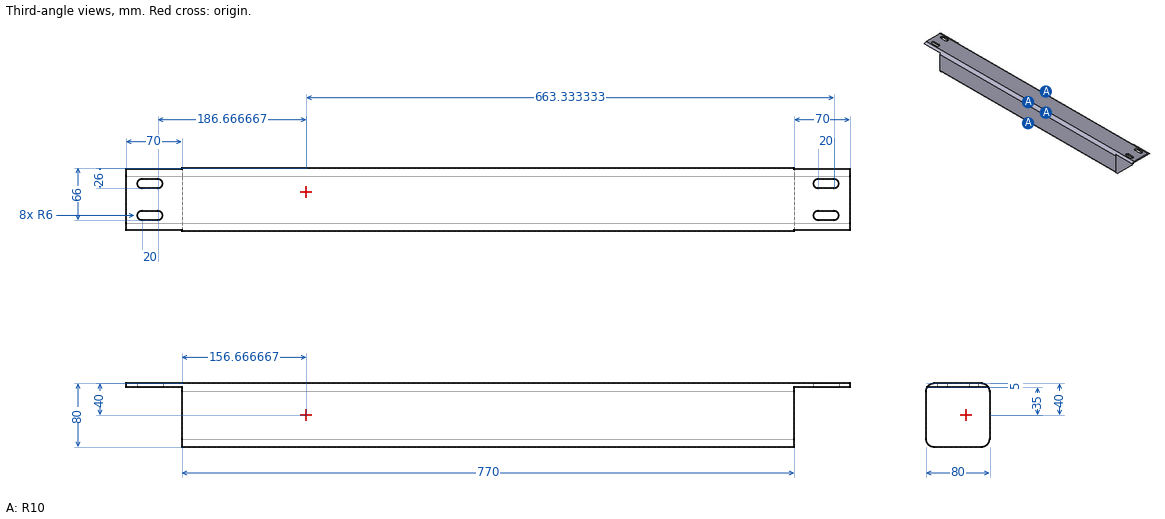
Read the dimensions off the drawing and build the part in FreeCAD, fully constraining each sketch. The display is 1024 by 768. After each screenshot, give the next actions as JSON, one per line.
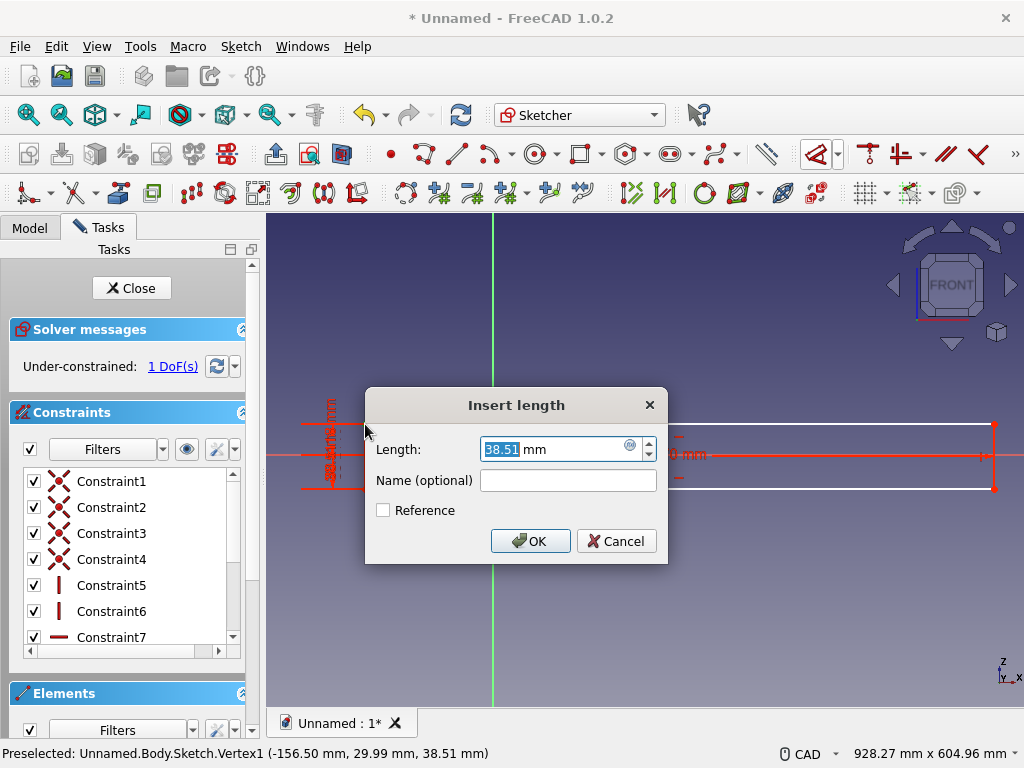
{"action": "type", "text": "40"}
{"action": "key", "text": "Return"}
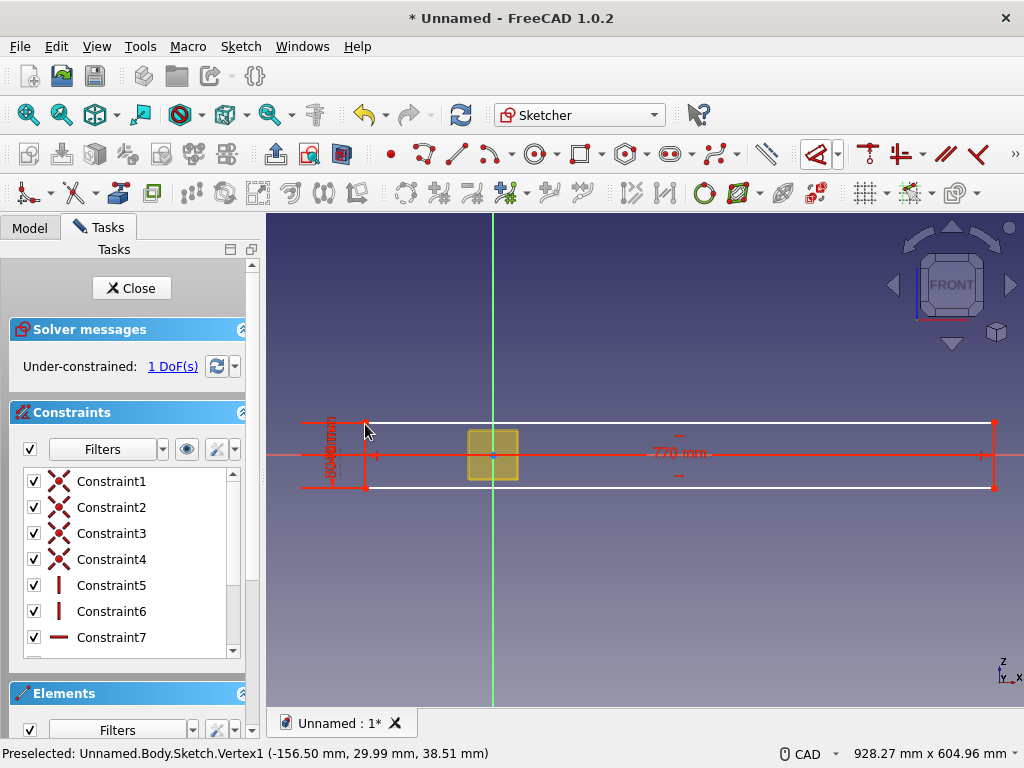
{"action": "left_click", "coordinate": [365, 423]}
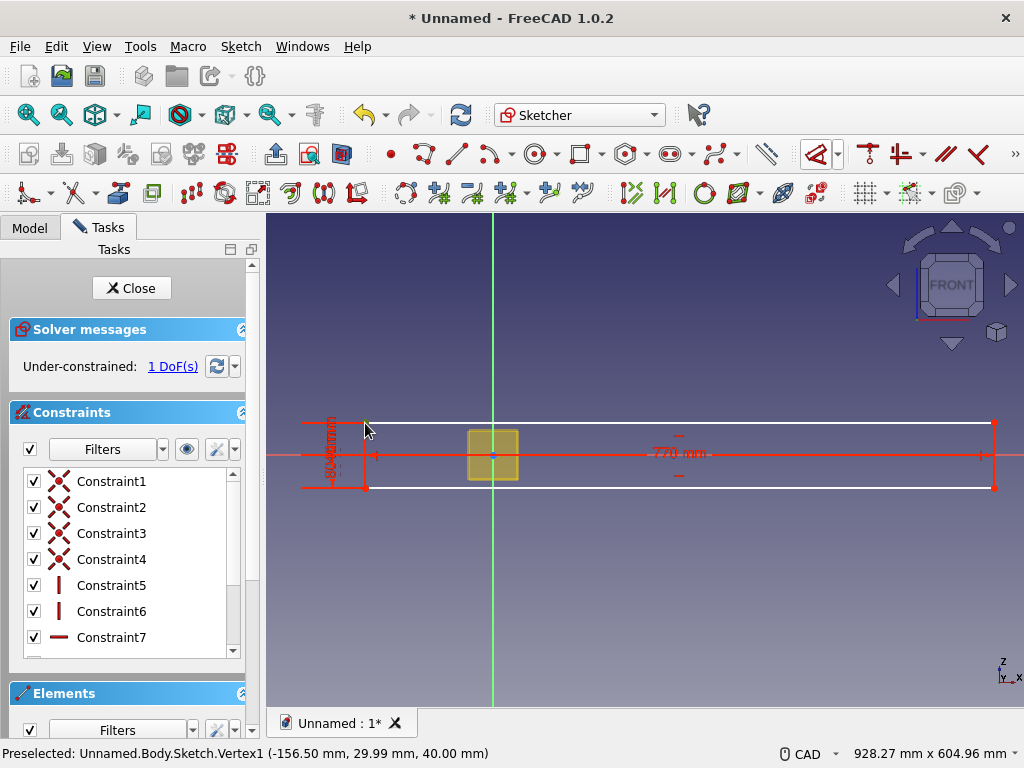
{"action": "left_click", "coordinate": [838, 154]}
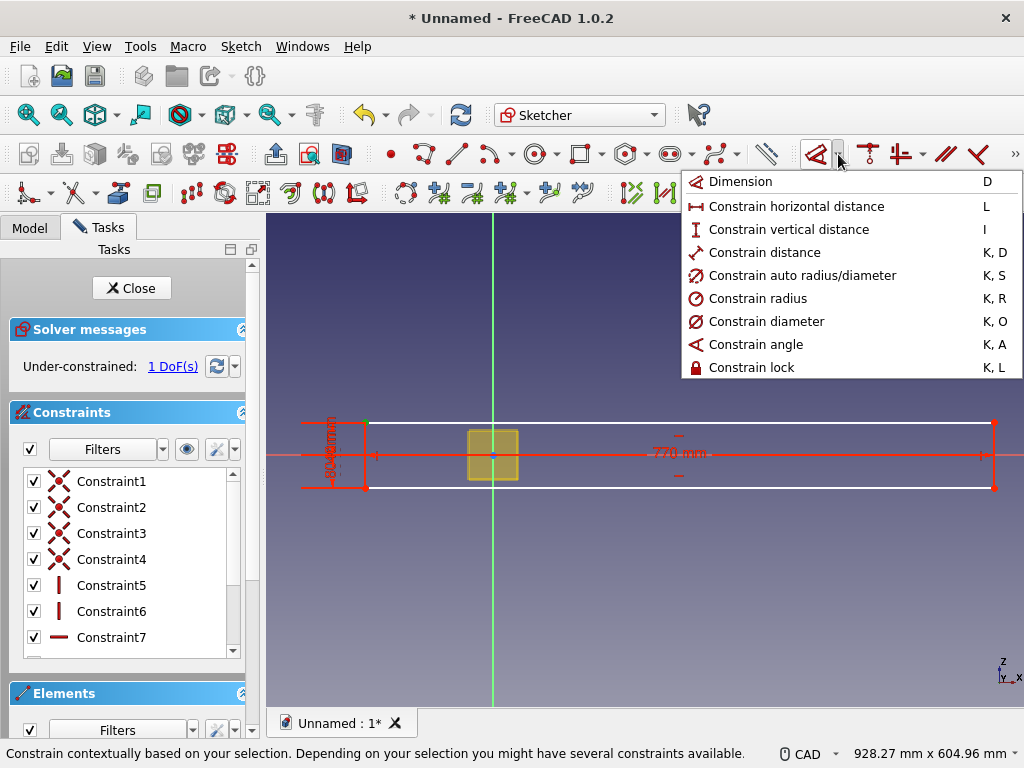
{"action": "left_click", "coordinate": [852, 206]}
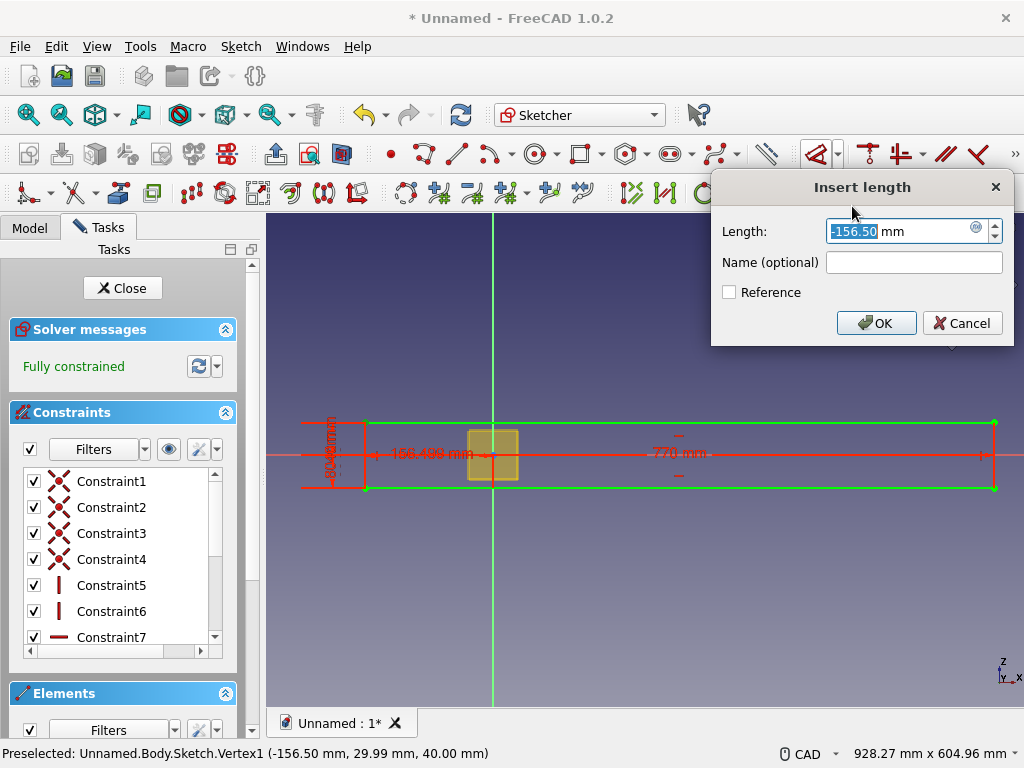
{"action": "type", "text": "-156.666667"}
{"action": "key", "text": "Return"}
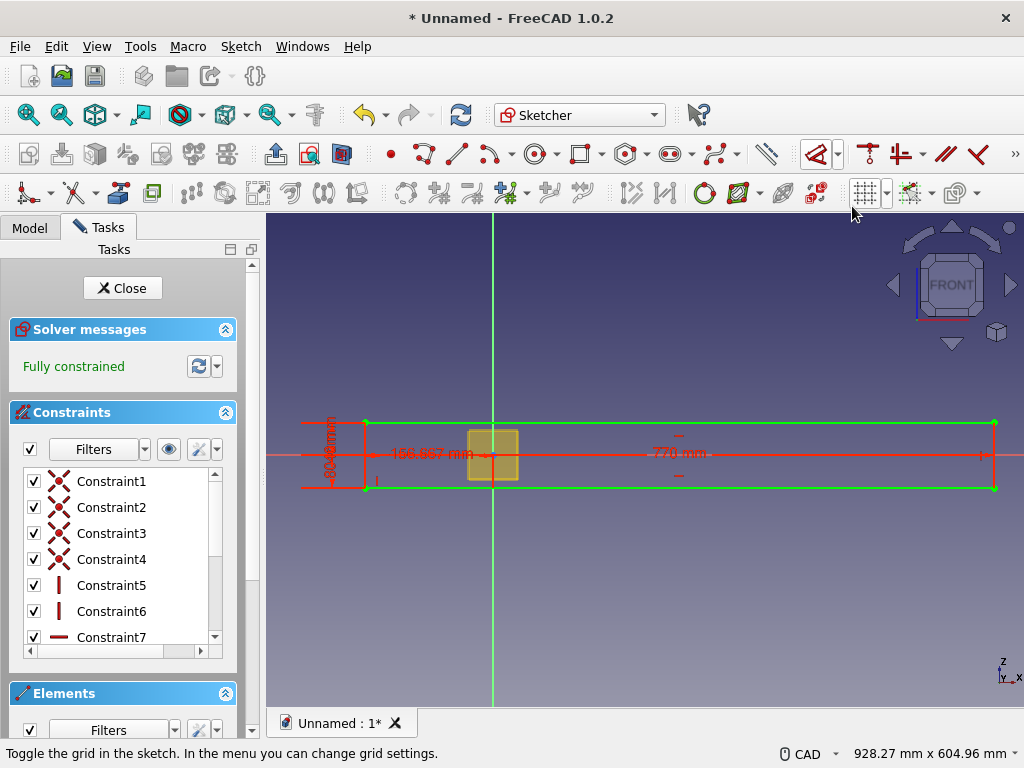
{"action": "left_click", "coordinate": [123, 288]}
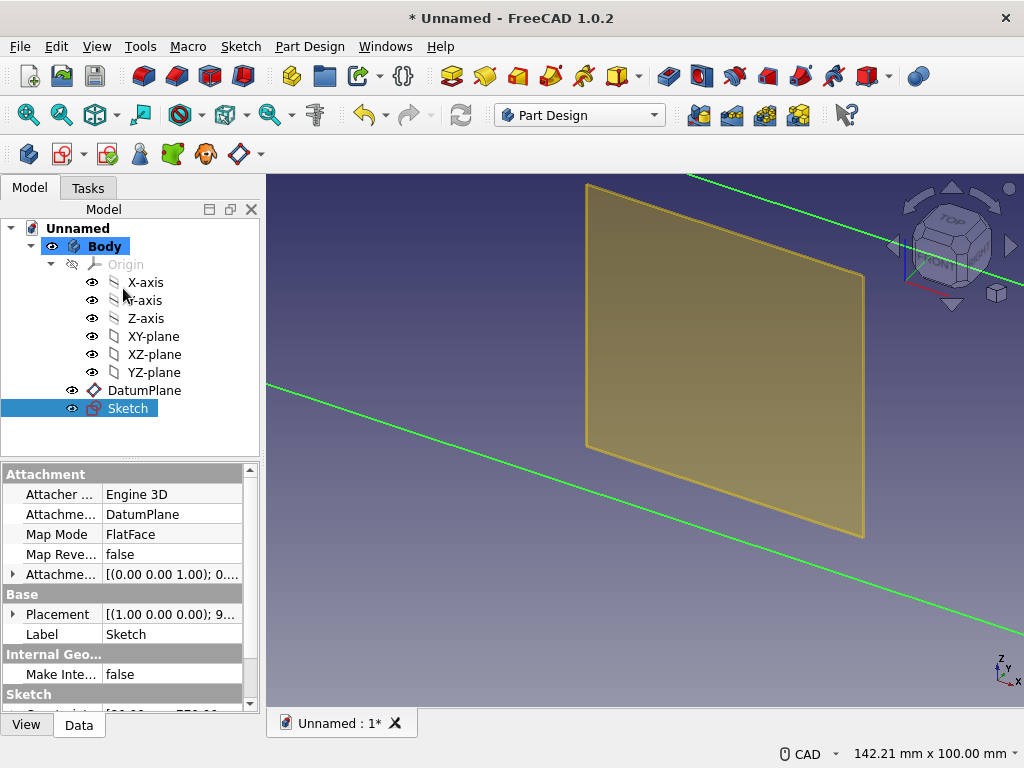
{"action": "left_click", "coordinate": [452, 76]}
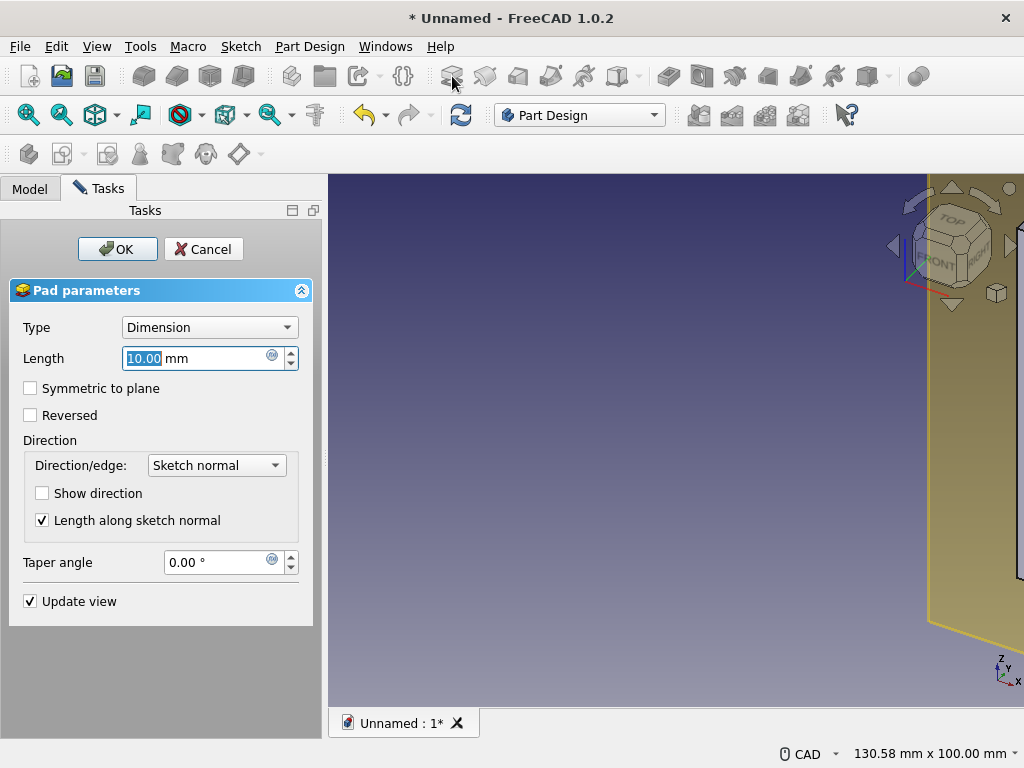
{"action": "type", "text": "80"}
{"action": "key", "text": "Tab"}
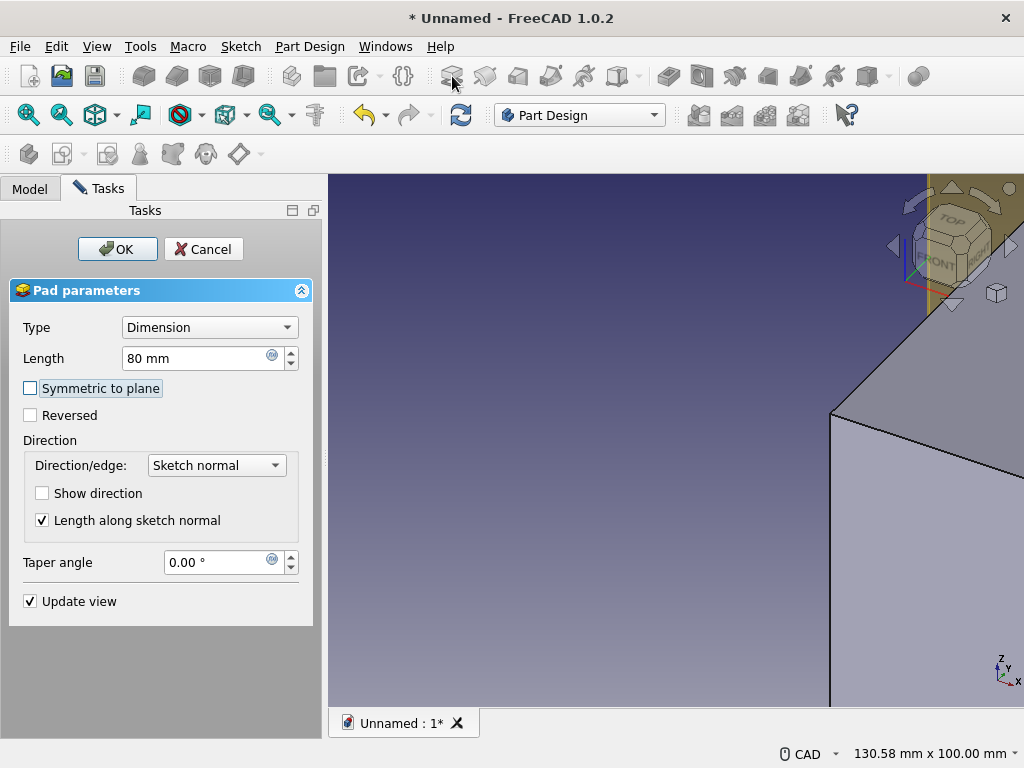
{"action": "left_click", "coordinate": [118, 249]}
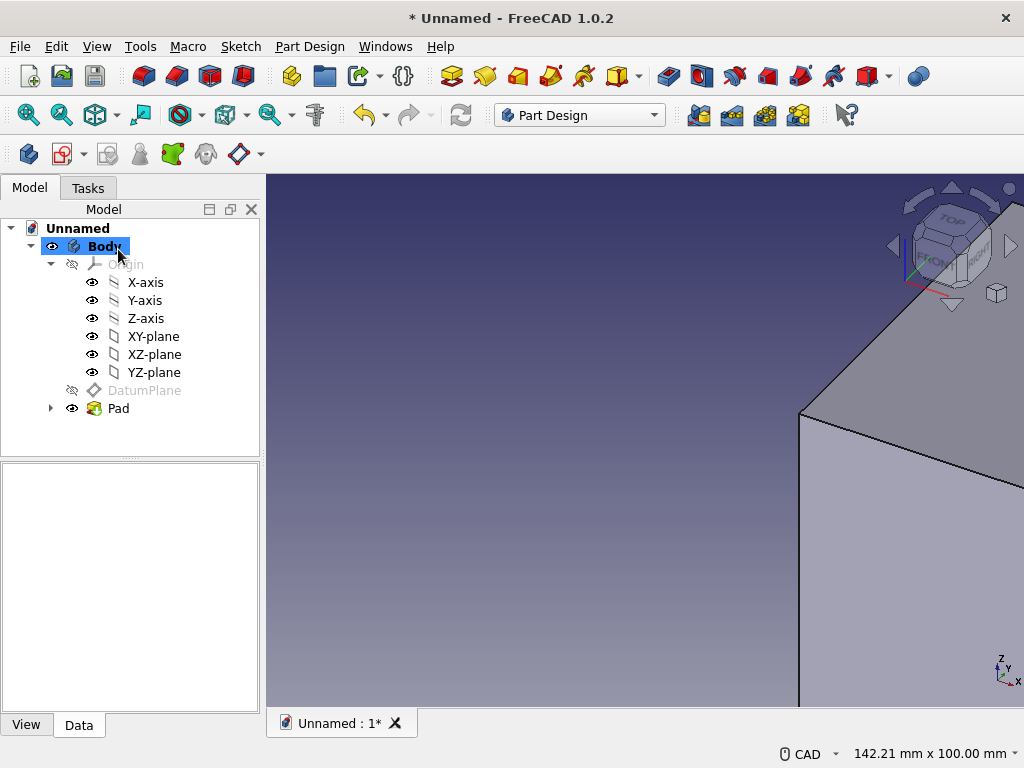
{"action": "left_click", "coordinate": [29, 116]}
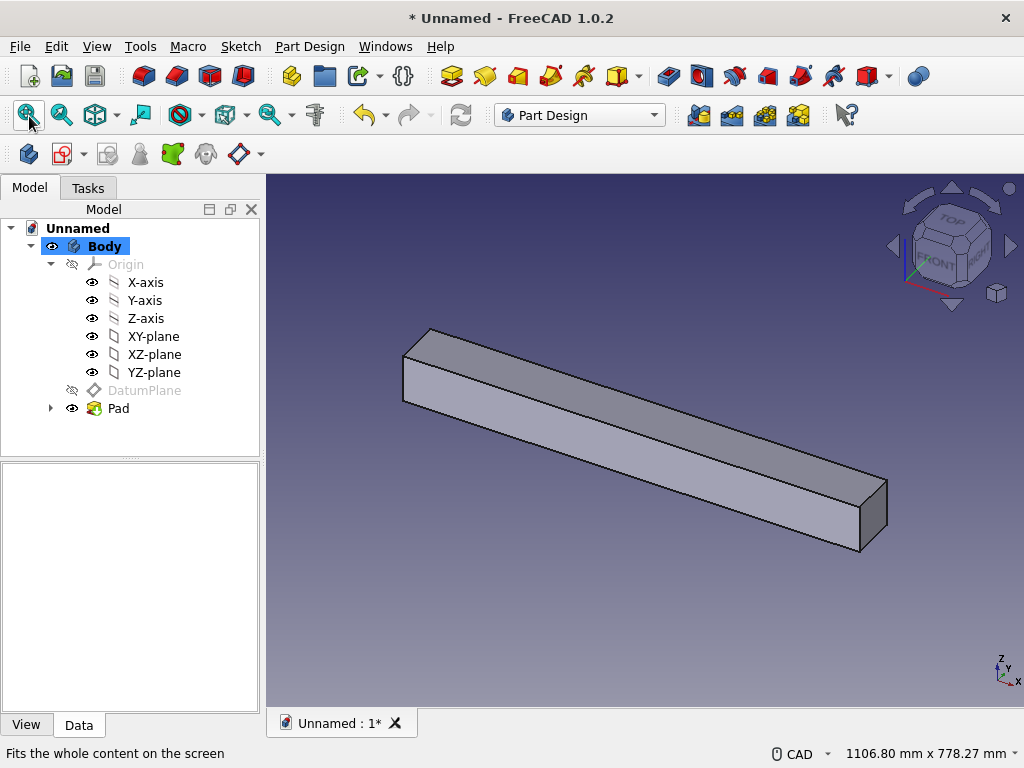
{"action": "key", "text": "6"}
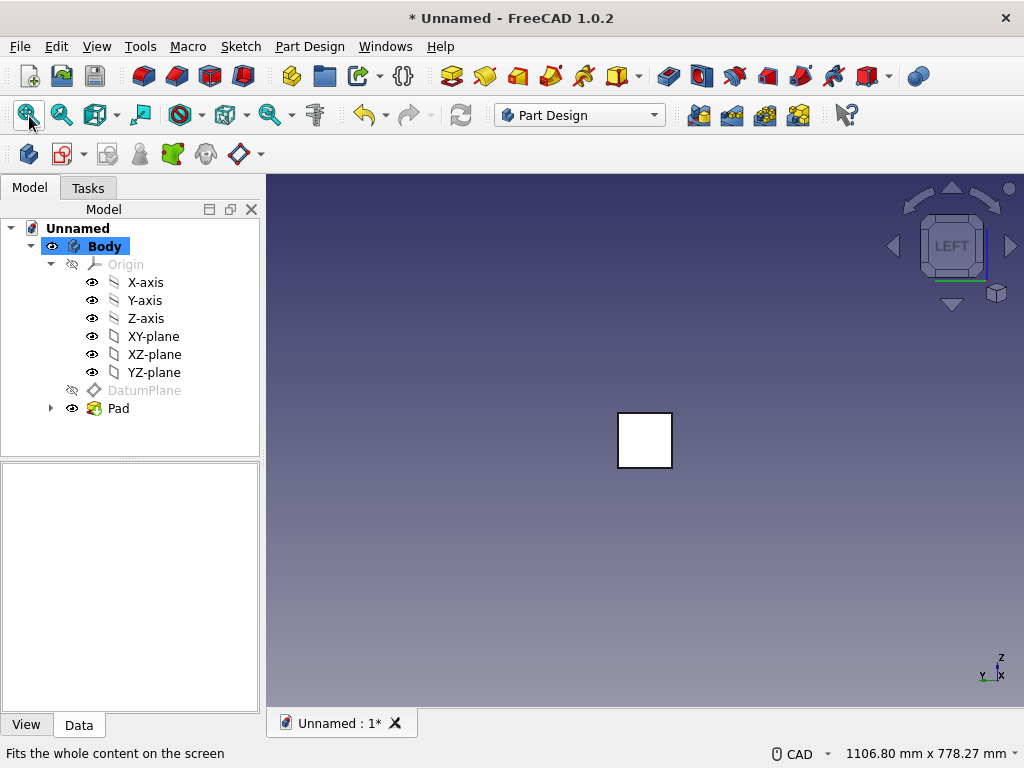
{"action": "left_click", "coordinate": [29, 116]}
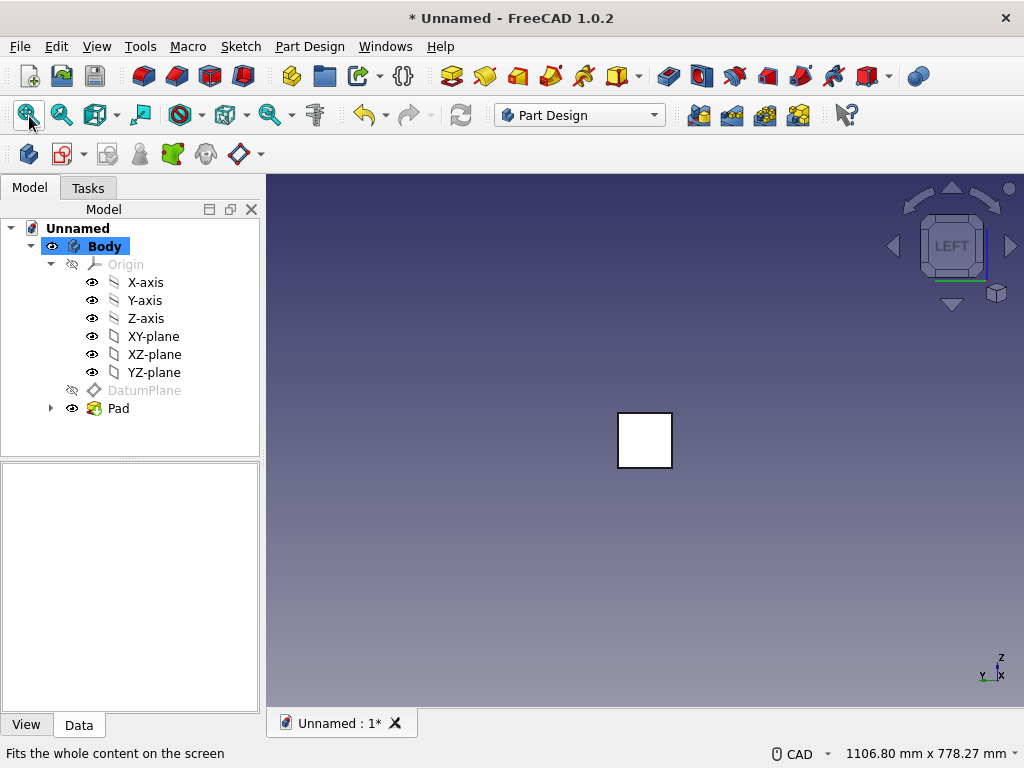
{"action": "left_click", "coordinate": [645, 439]}